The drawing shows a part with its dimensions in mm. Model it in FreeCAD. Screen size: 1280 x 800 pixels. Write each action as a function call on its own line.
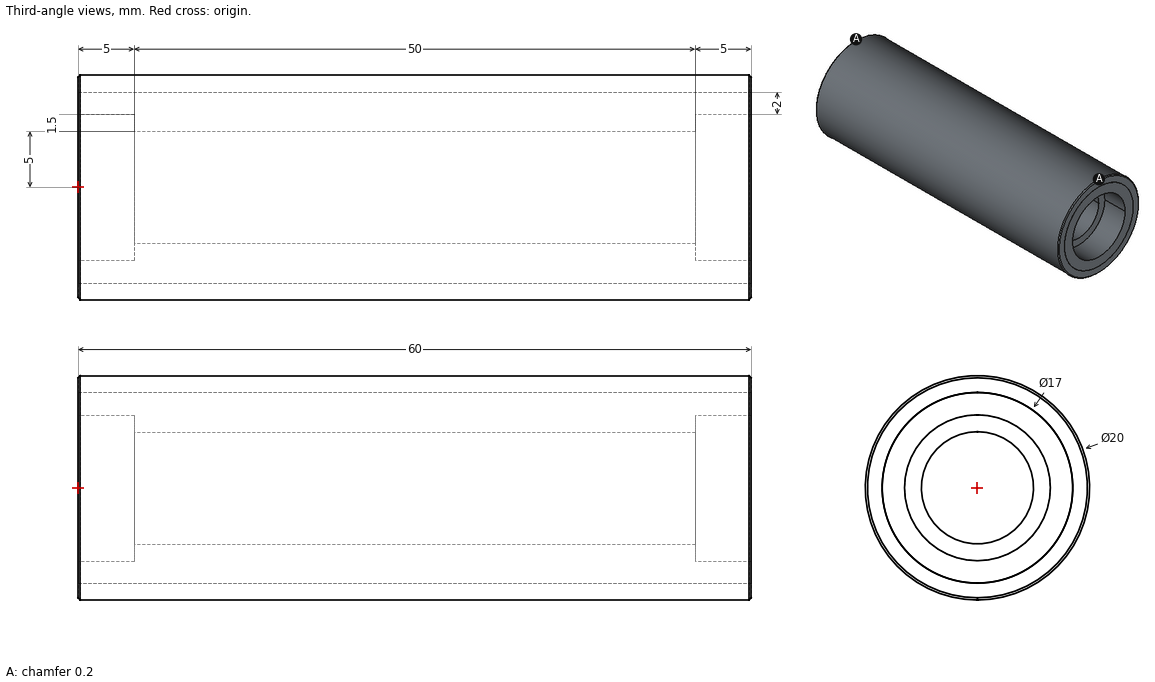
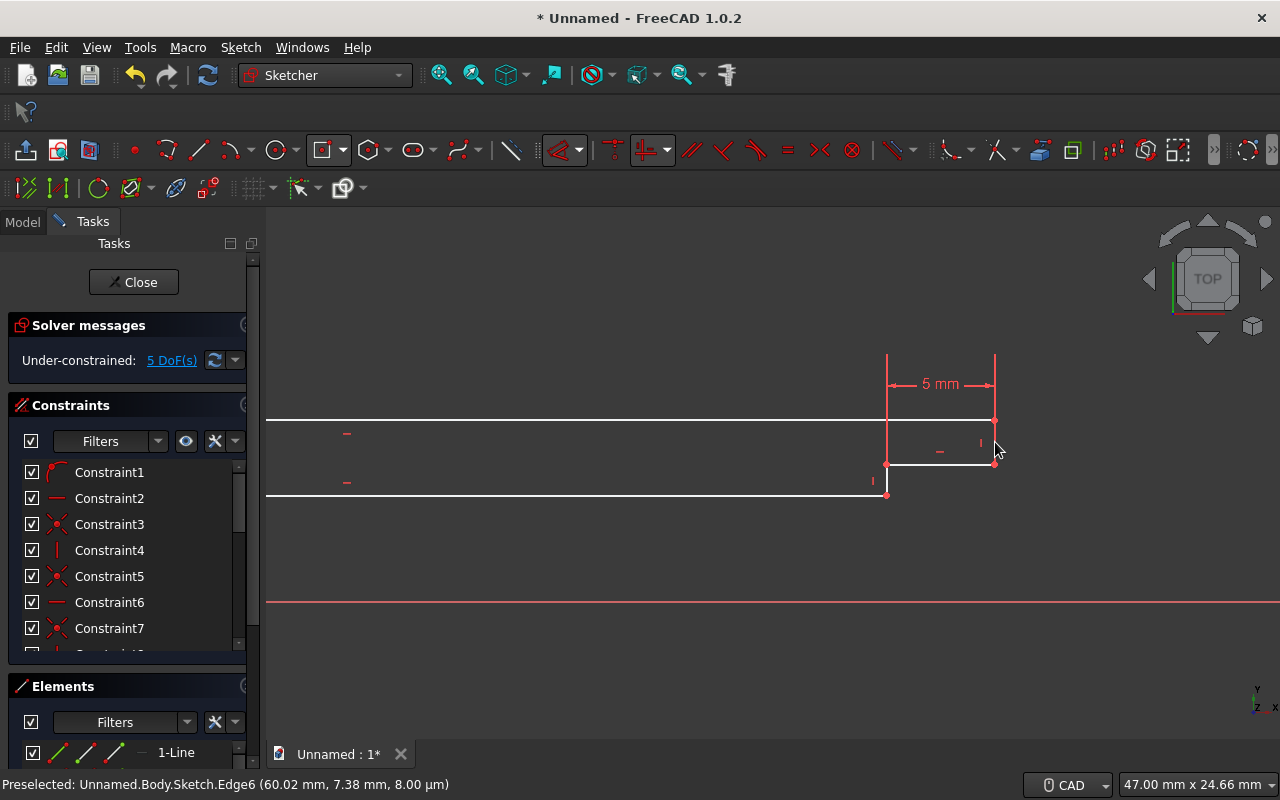
key(i)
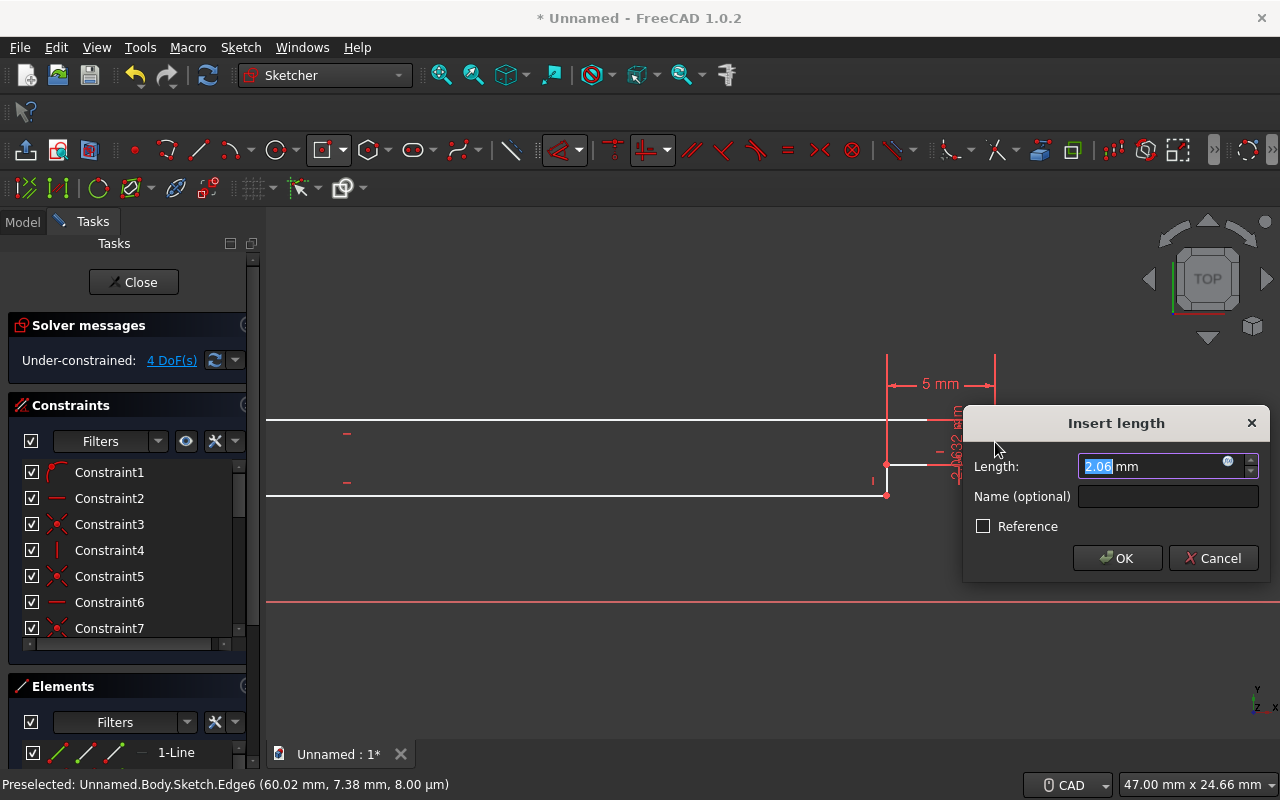
text(2)
key(Return)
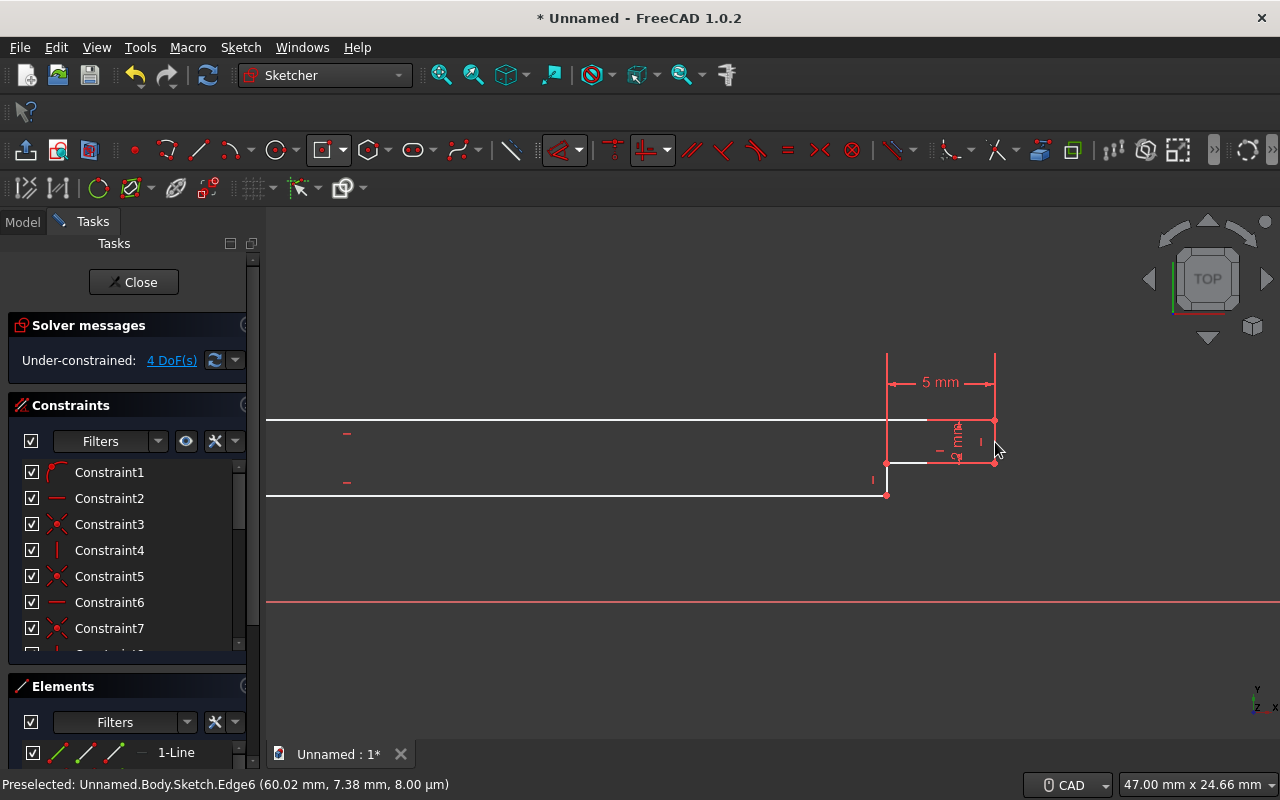
scroll(996, 442, down, 4)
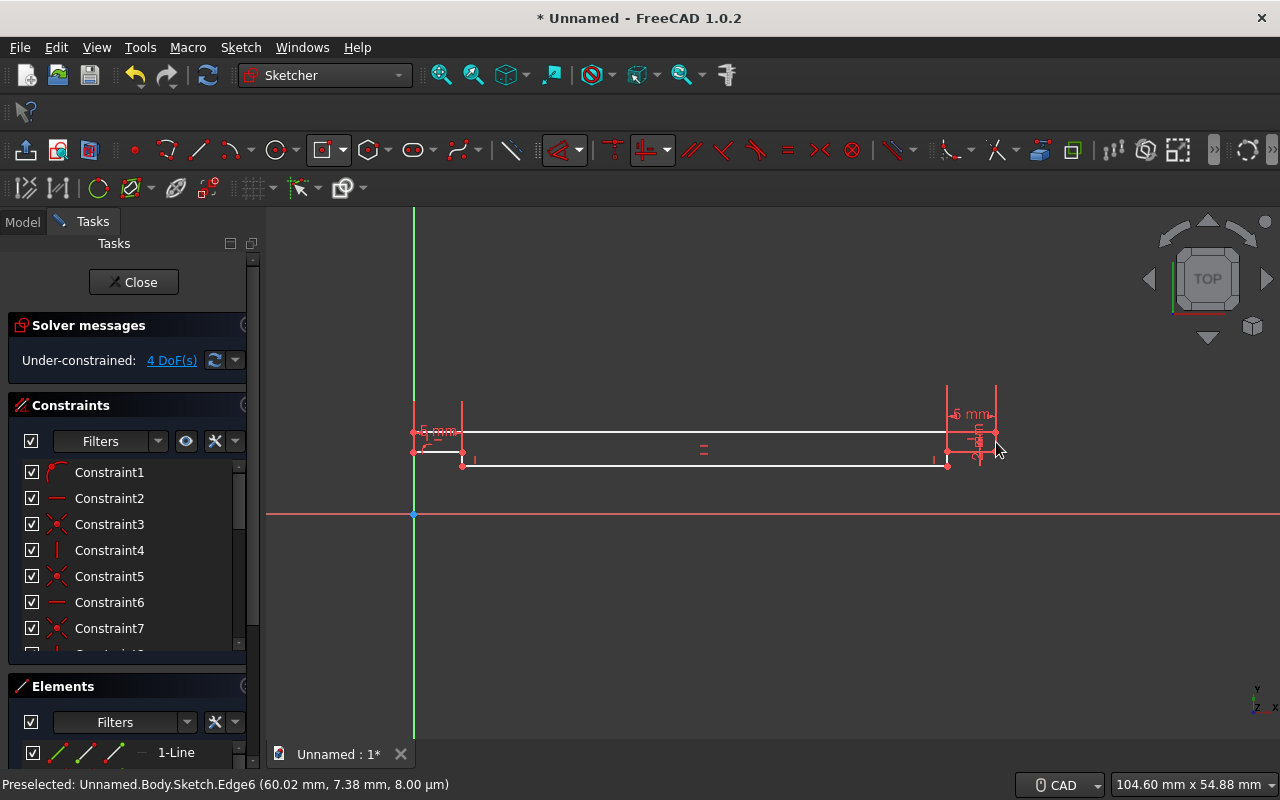
scroll(414, 438, up, 5)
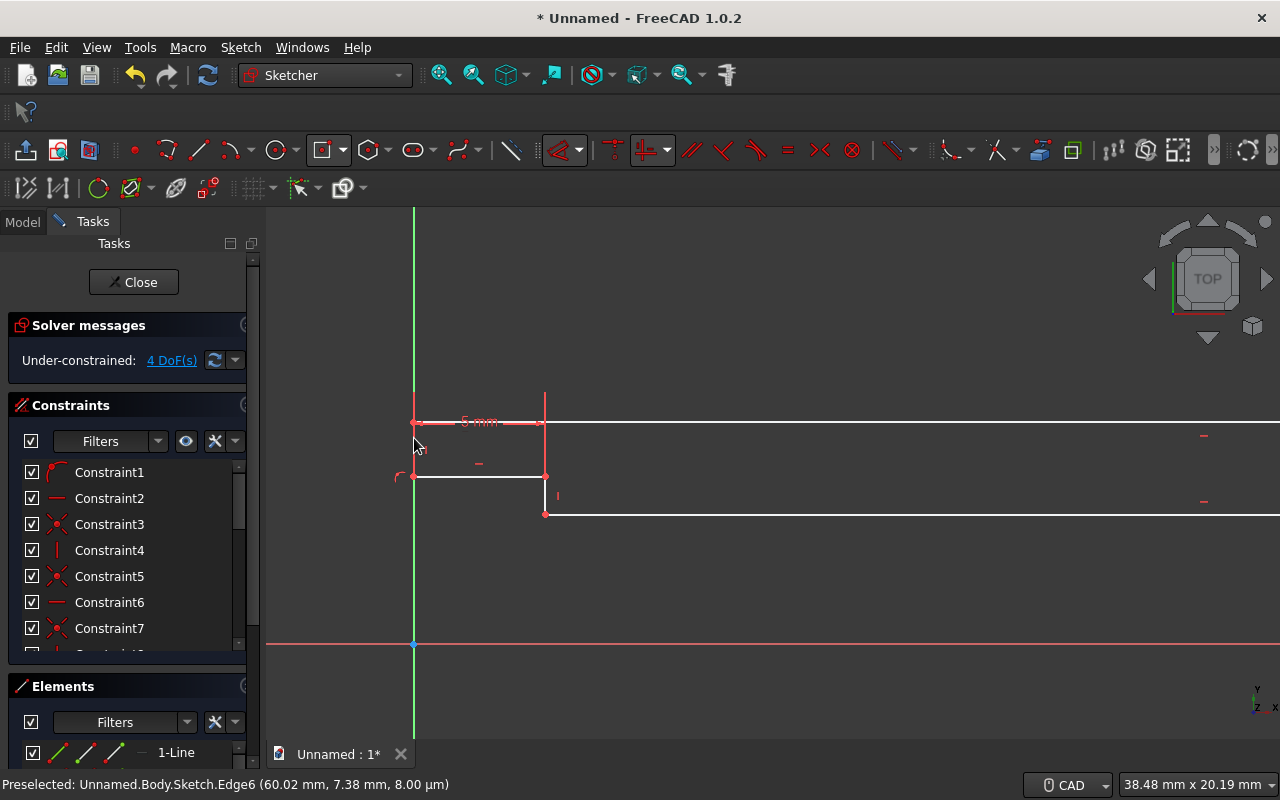
click(414, 438)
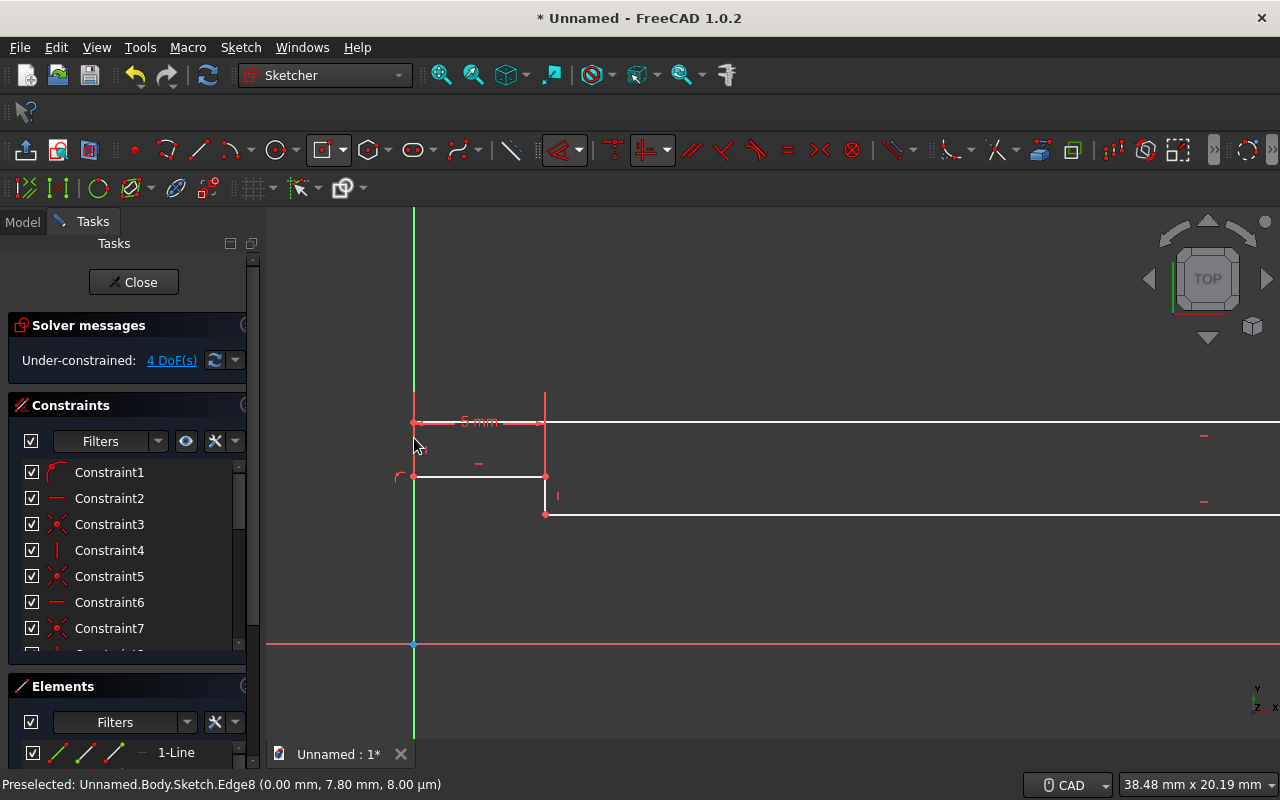
click(582, 150)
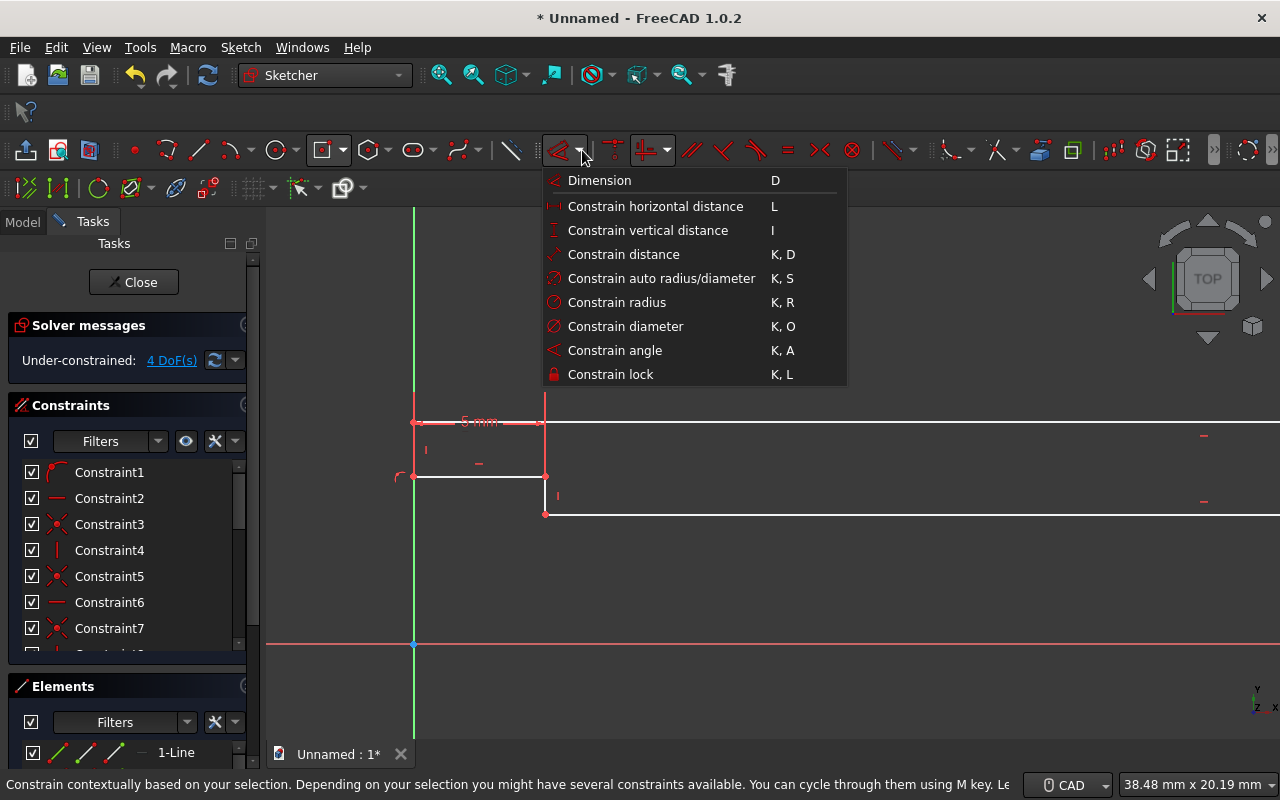
click(695, 230)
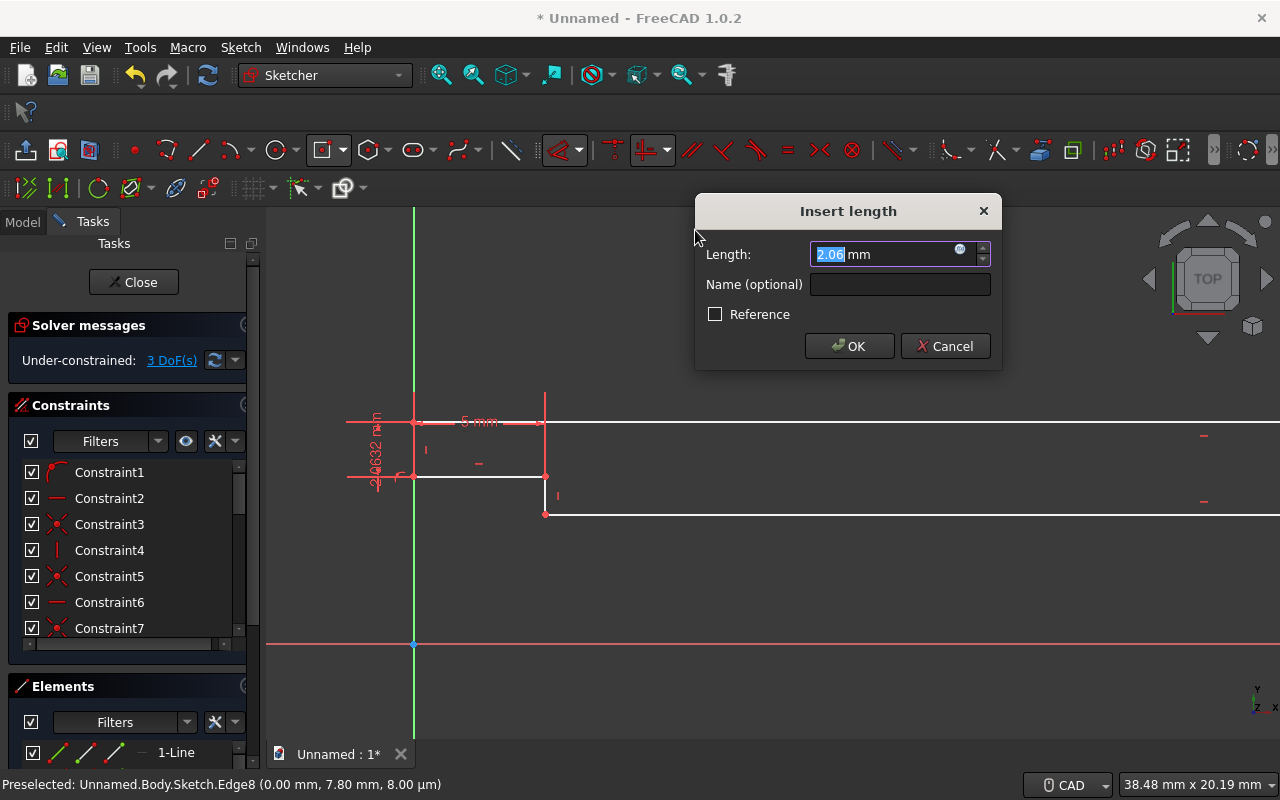
text(2)
key(Return)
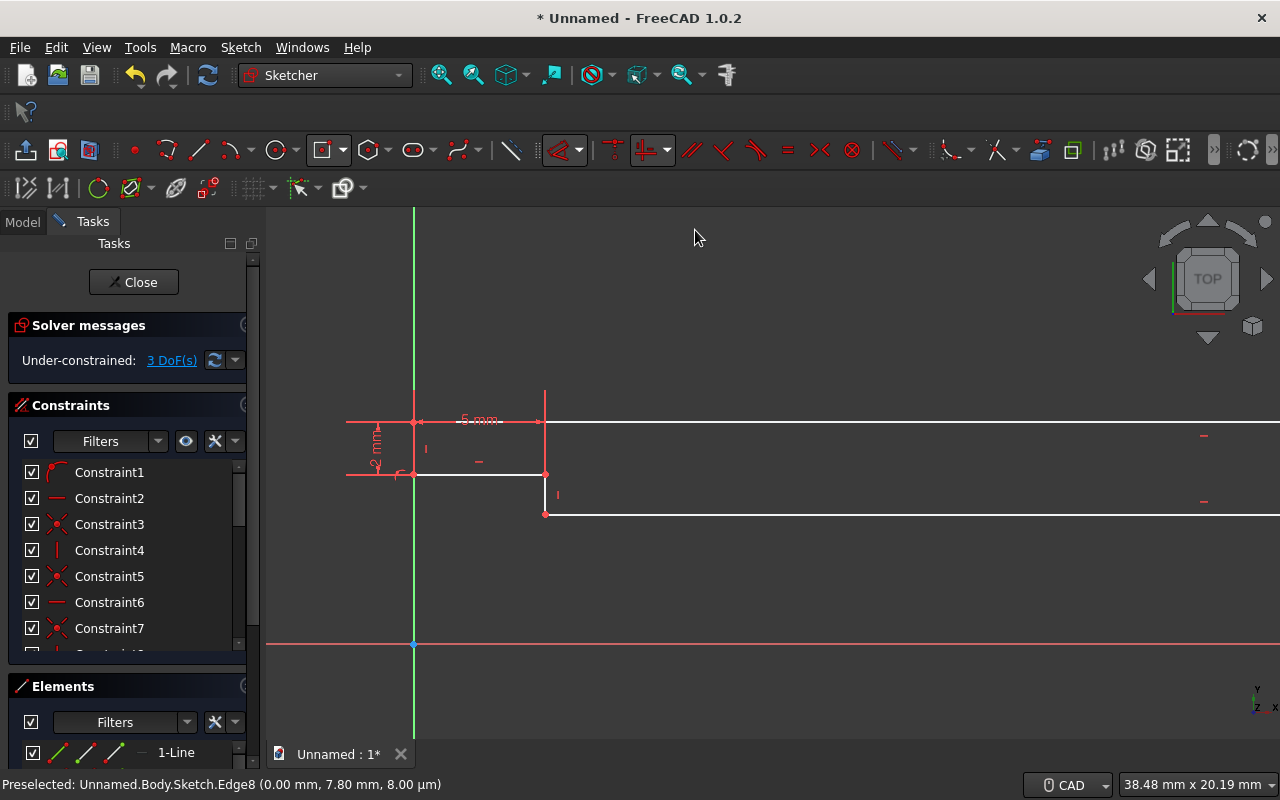
click(941, 515)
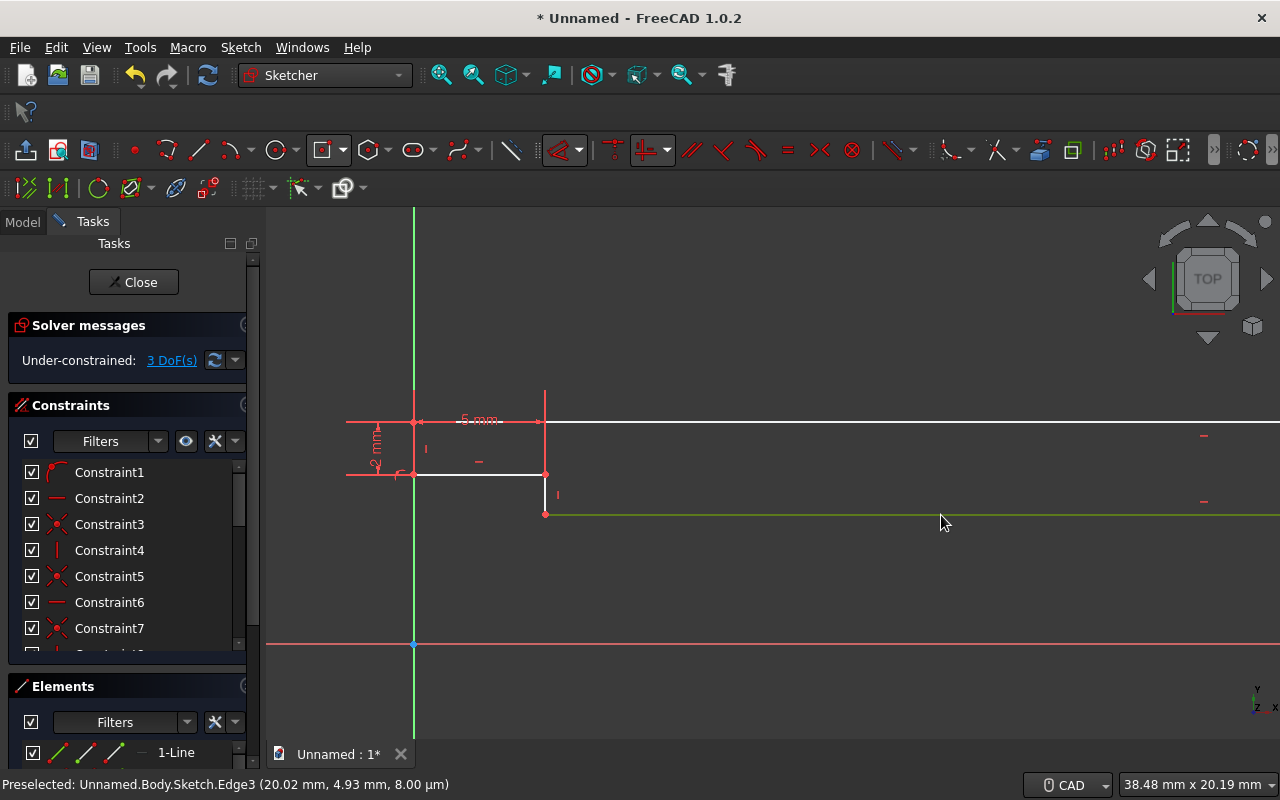
key(l)